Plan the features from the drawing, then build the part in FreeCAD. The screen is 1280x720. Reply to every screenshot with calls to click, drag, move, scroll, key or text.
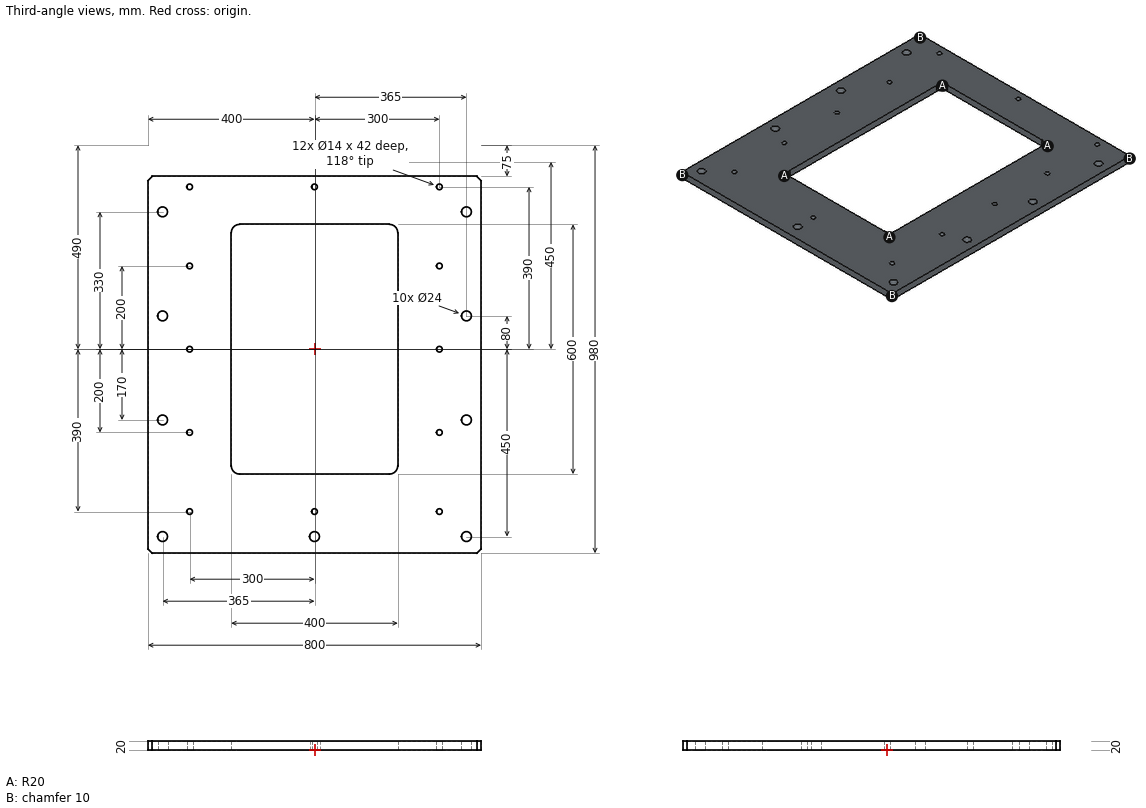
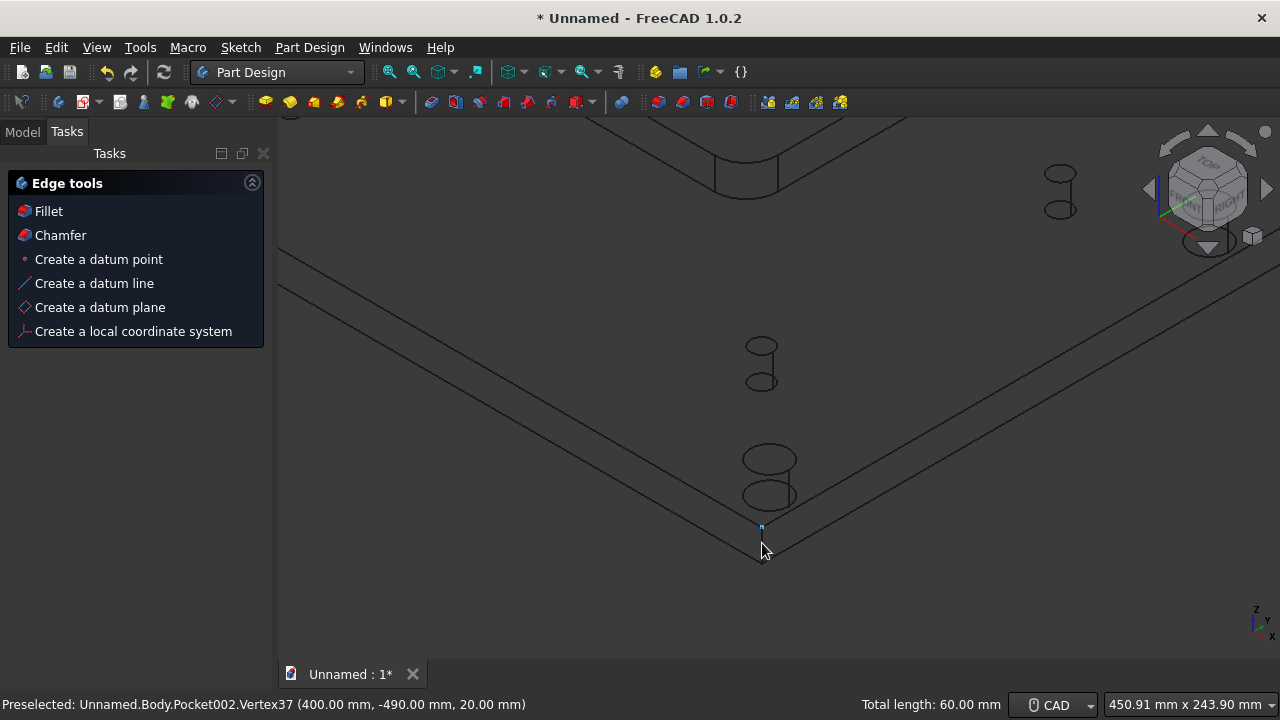
click(762, 545, ctrl)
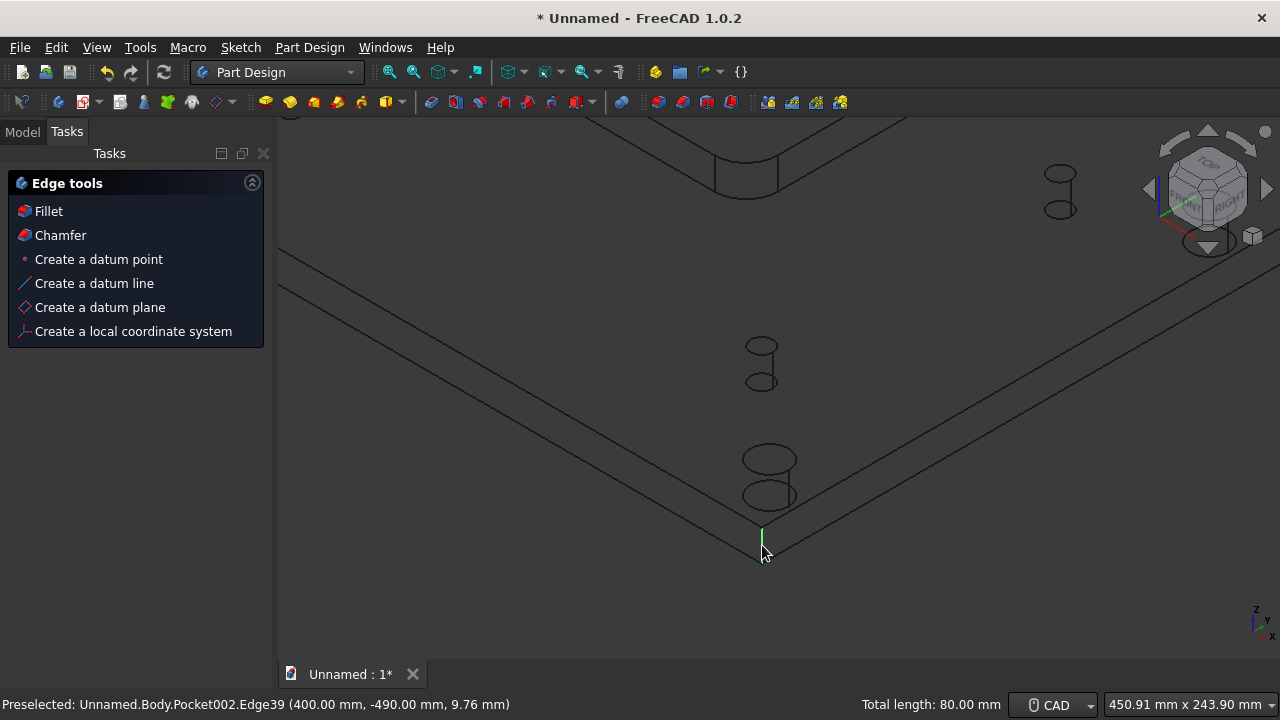
key(v)
key(1)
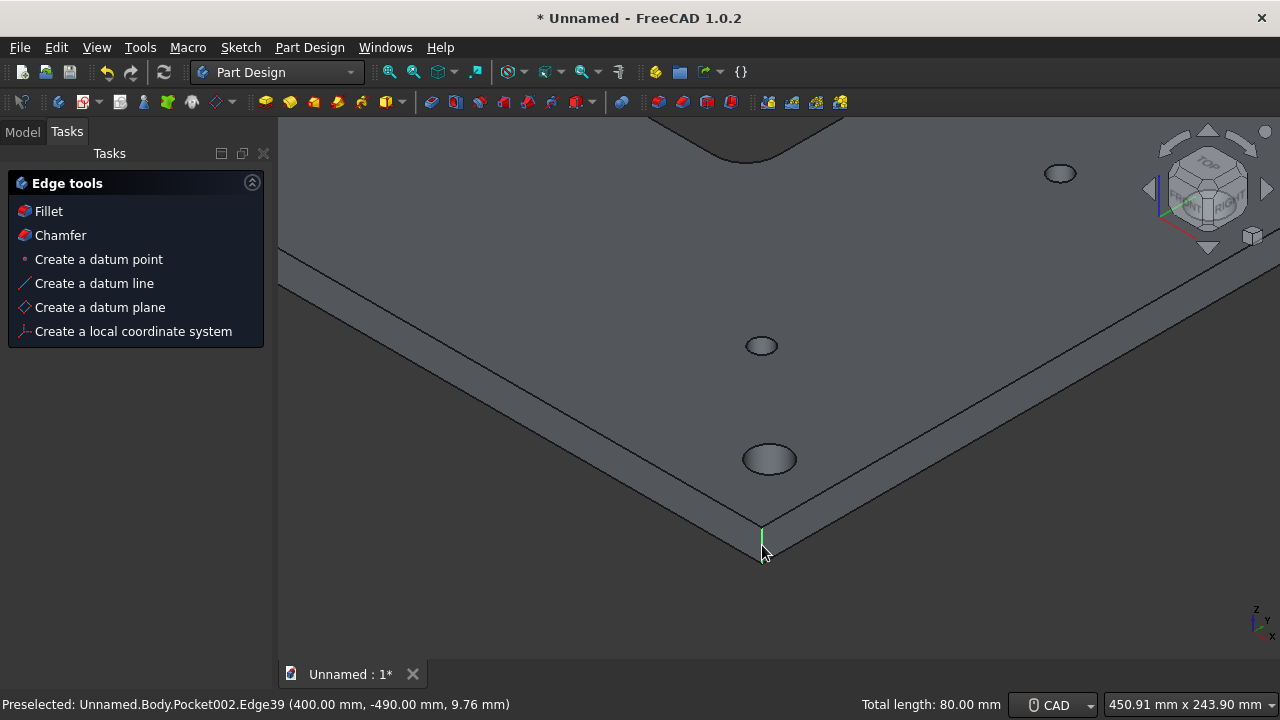
click(684, 102)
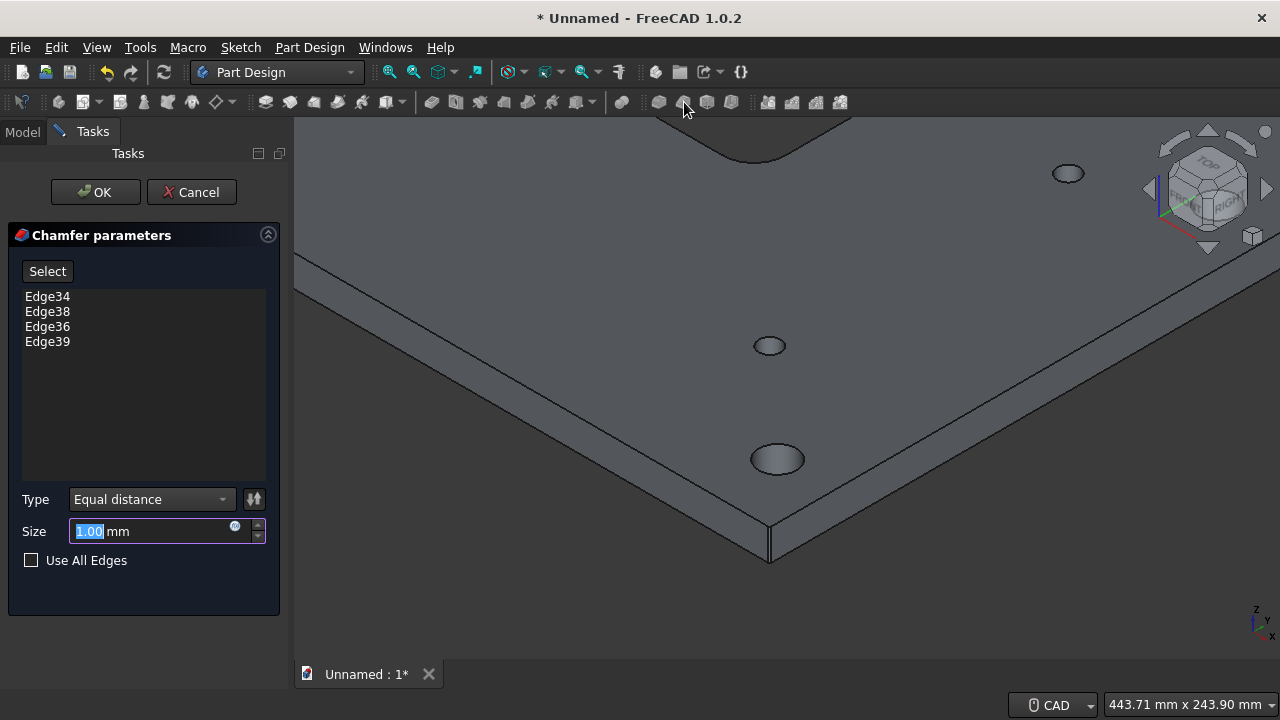
text(10)
key(Tab)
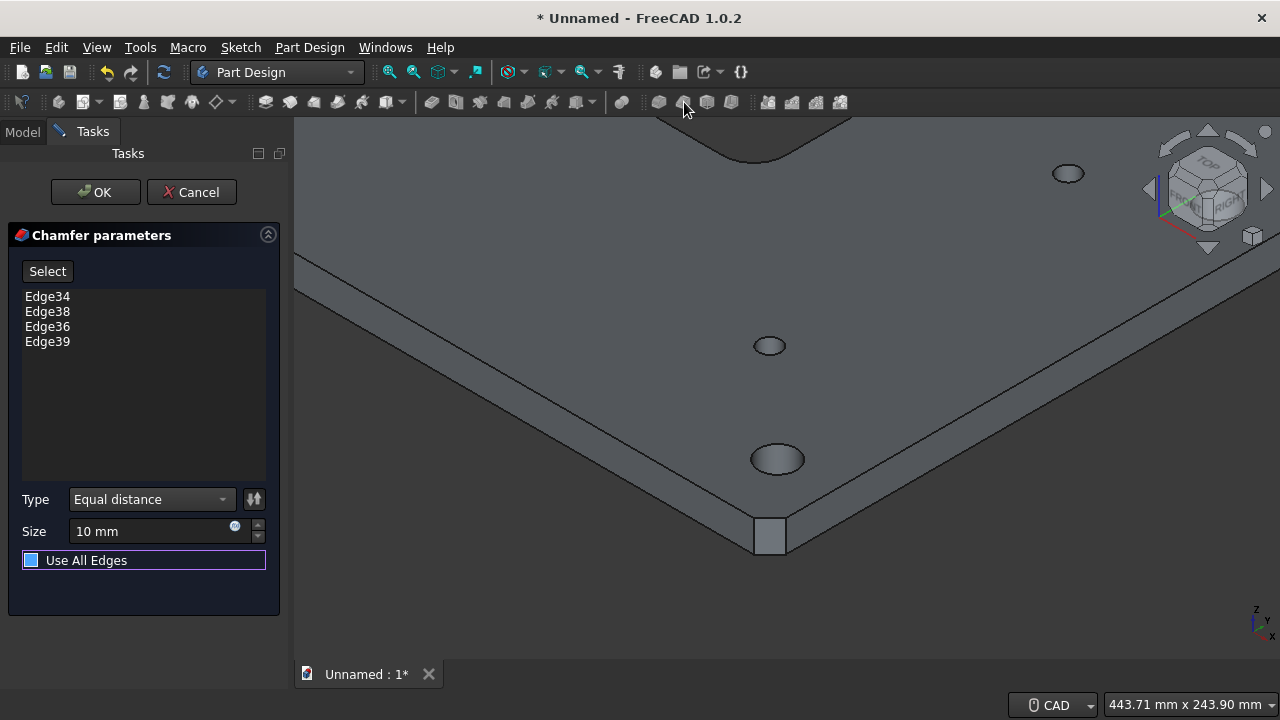
click(96, 192)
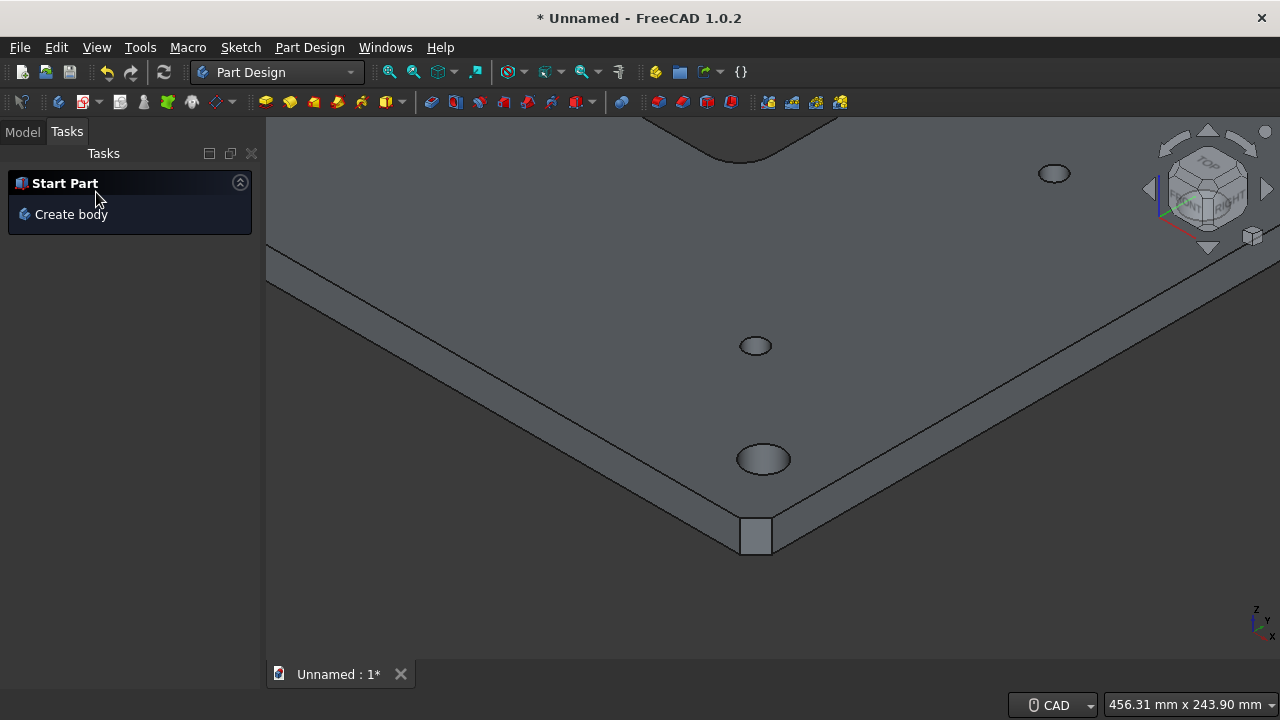
click(390, 72)